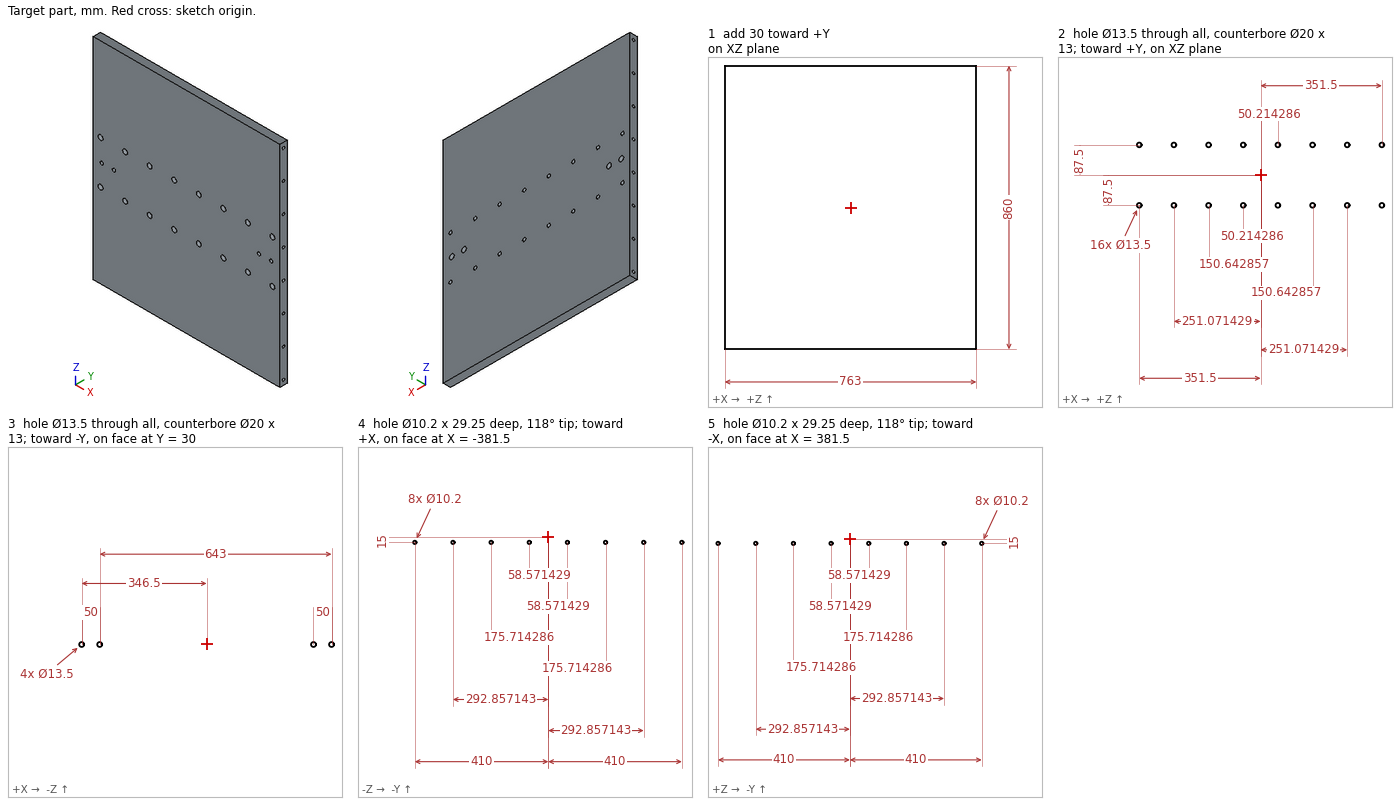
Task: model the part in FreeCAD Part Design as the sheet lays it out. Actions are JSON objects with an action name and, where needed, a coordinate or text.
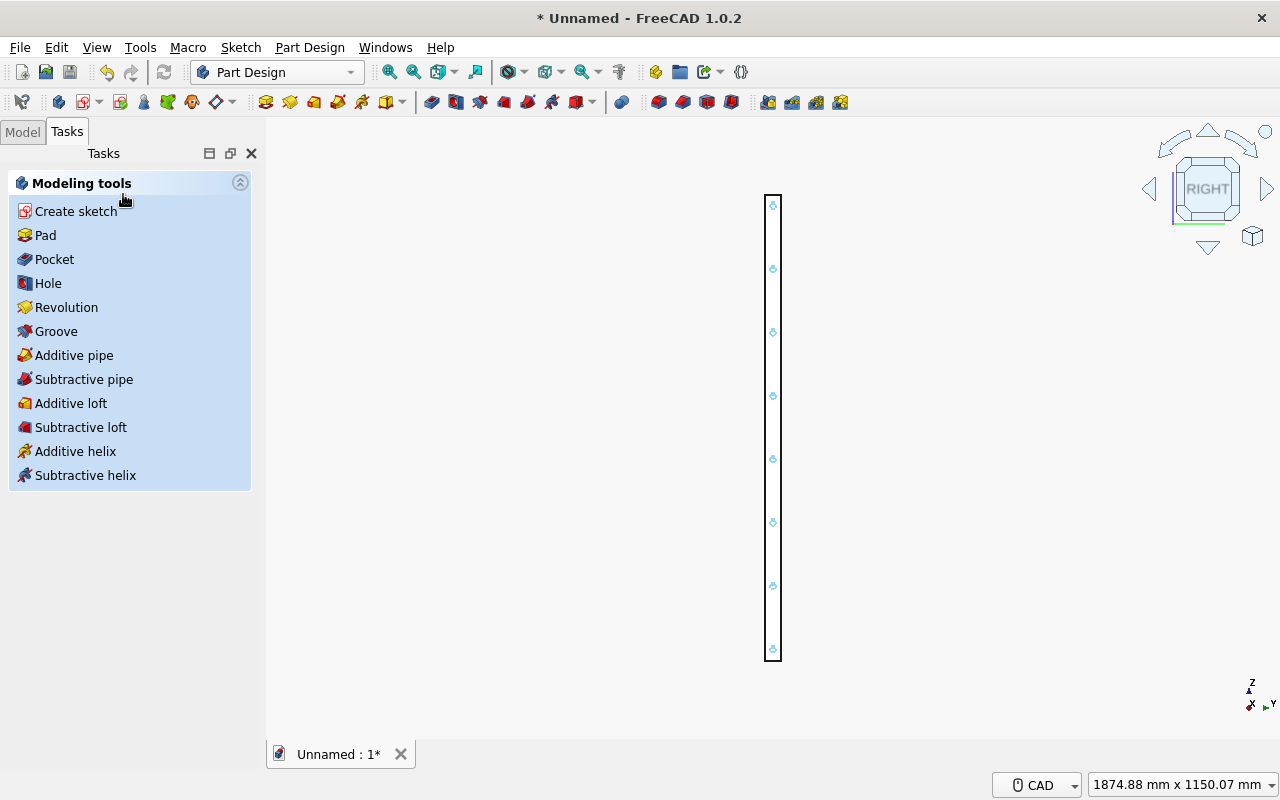
{"action": "left_click", "coordinate": [456, 102]}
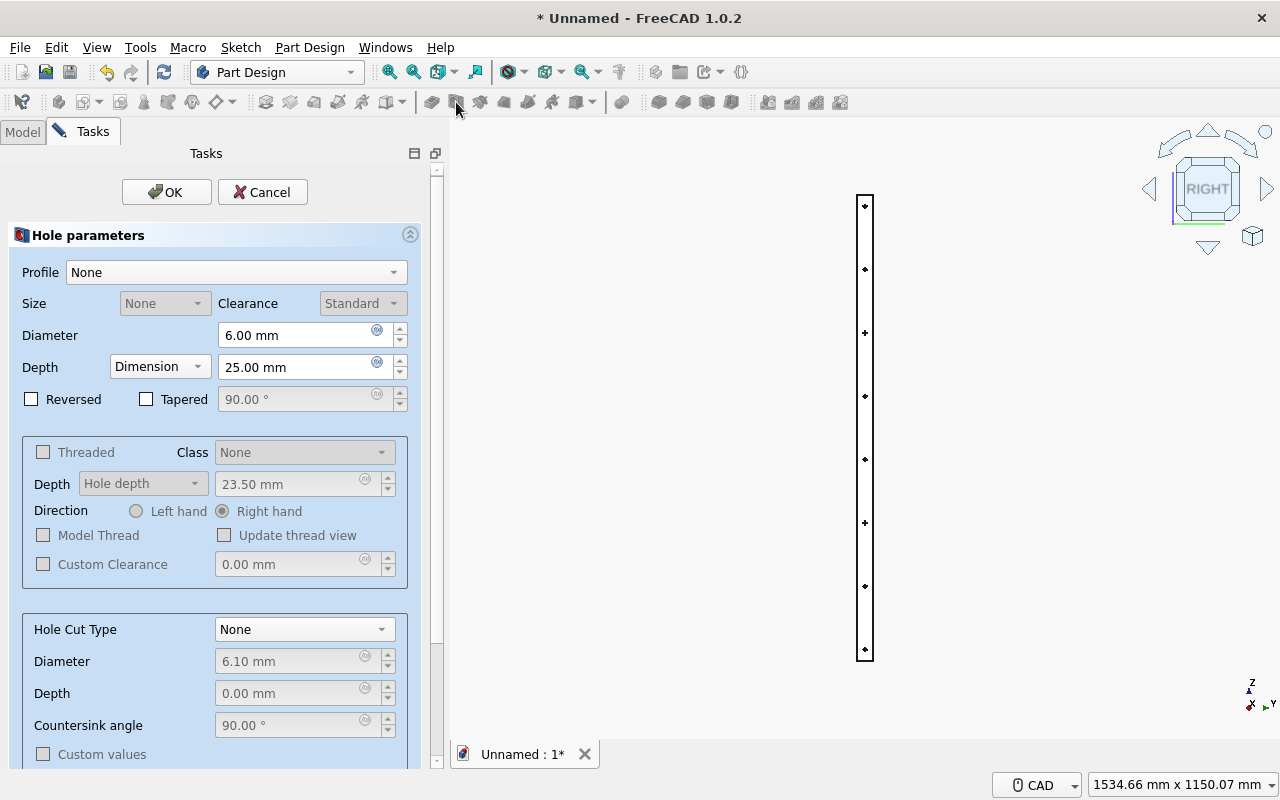
{"action": "triple_click", "coordinate": [305, 335]}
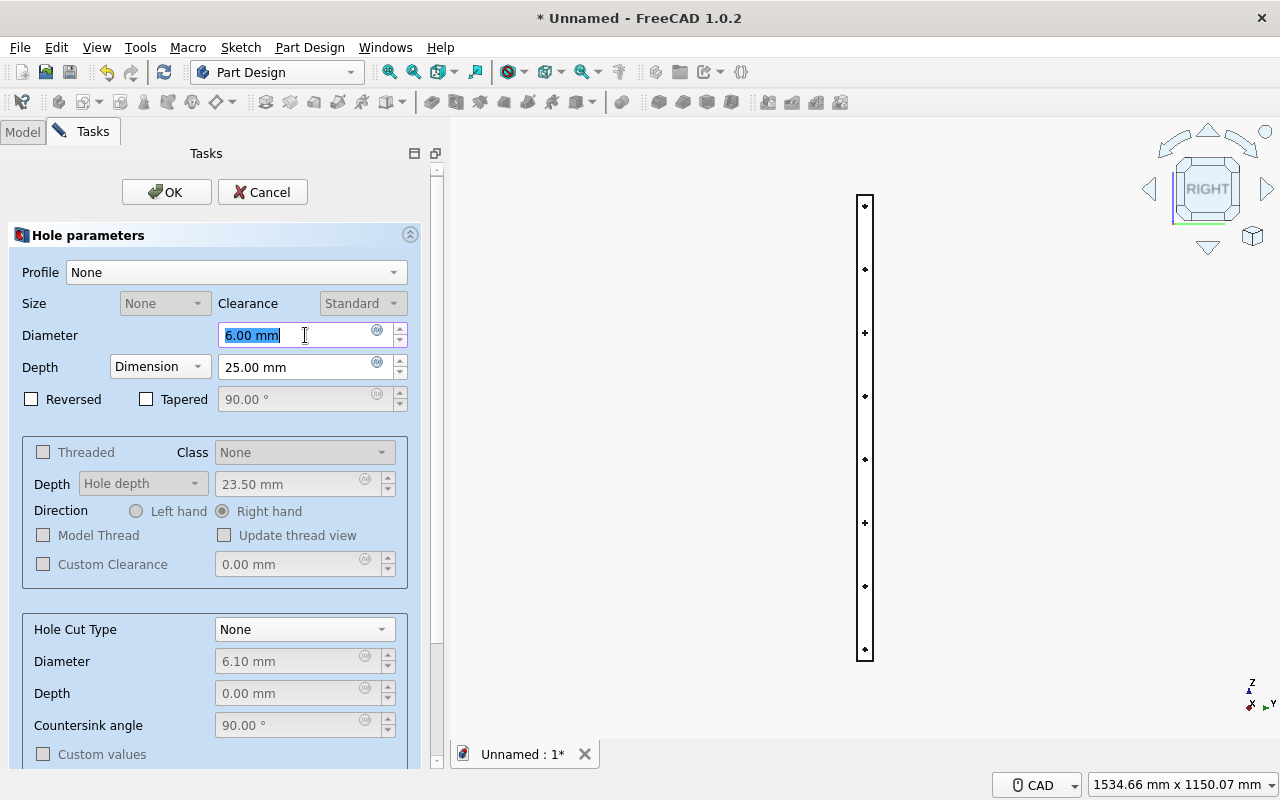
{"action": "type", "text": "10.2"}
{"action": "key", "text": "Tab"}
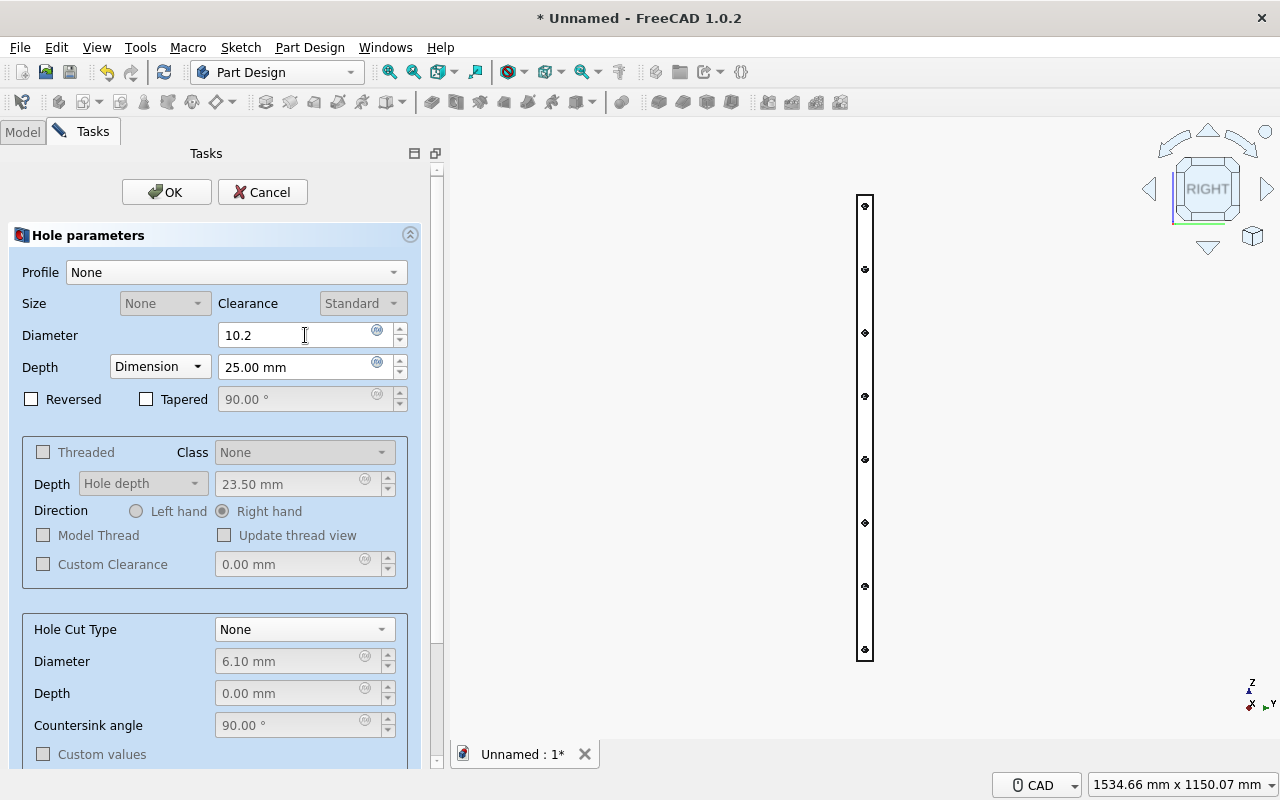
{"action": "triple_click", "coordinate": [305, 367]}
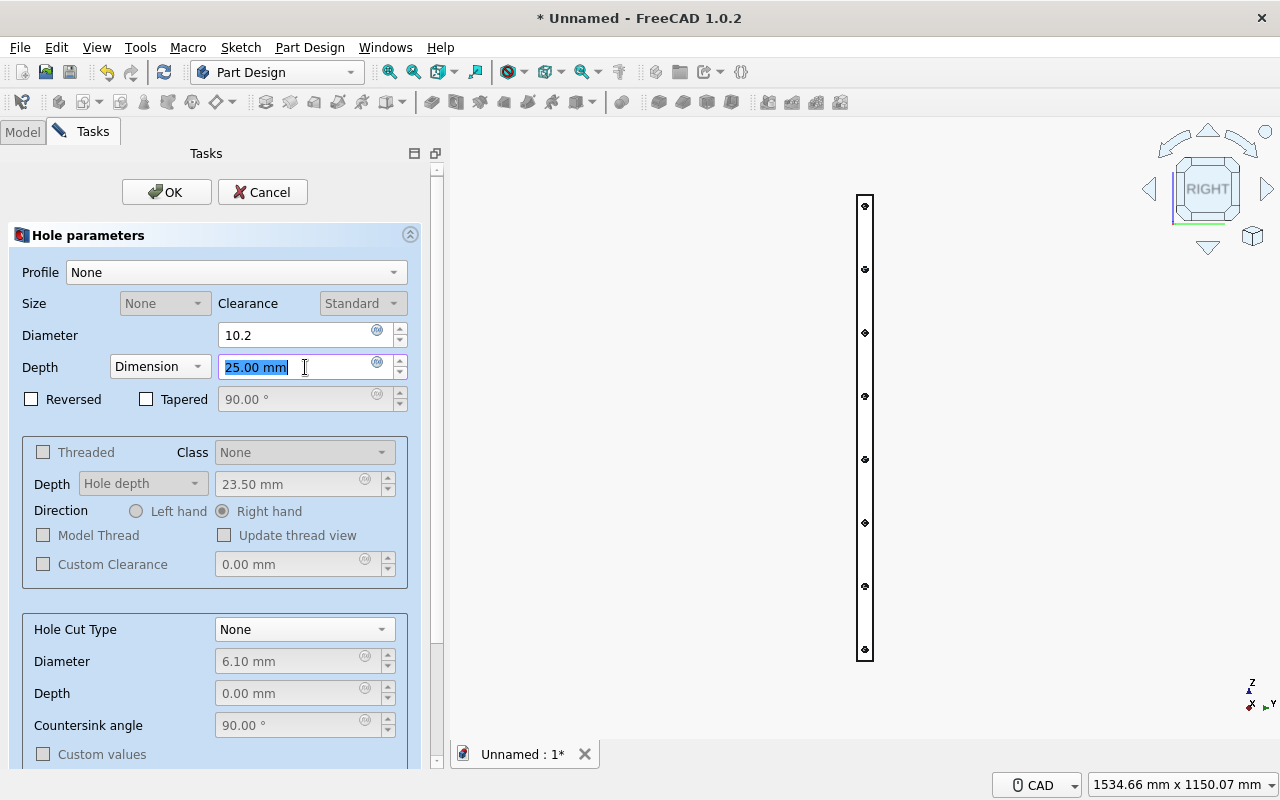
{"action": "type", "text": "29.25"}
{"action": "key", "text": "Tab"}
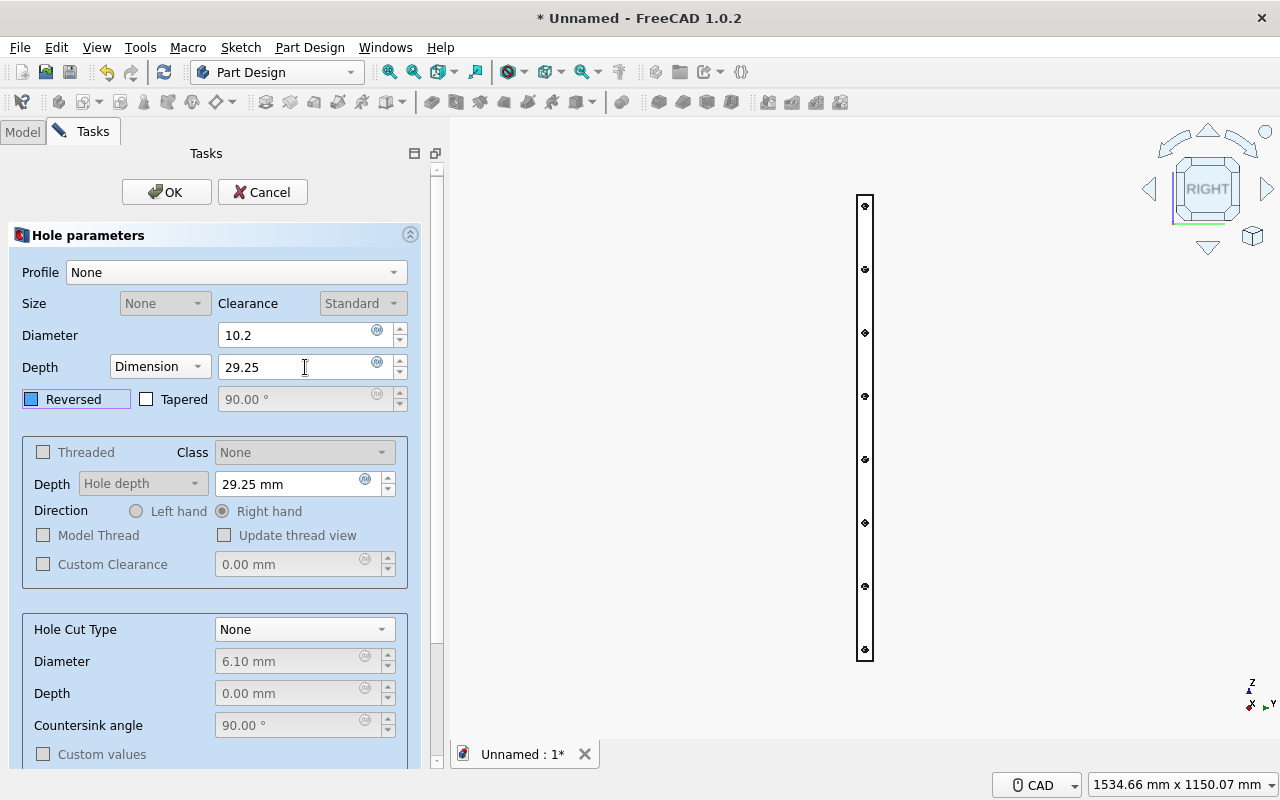
{"action": "left_click", "coordinate": [167, 192]}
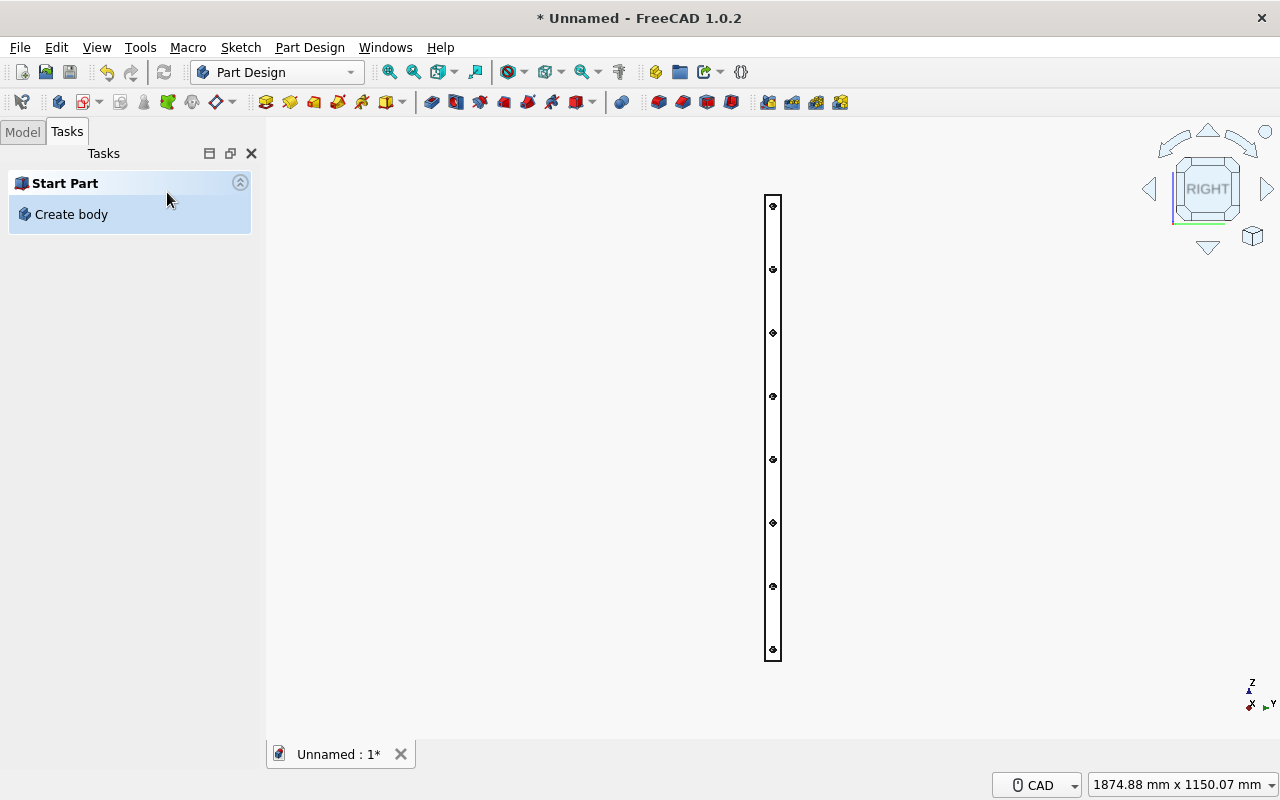
{"action": "key", "text": "0"}